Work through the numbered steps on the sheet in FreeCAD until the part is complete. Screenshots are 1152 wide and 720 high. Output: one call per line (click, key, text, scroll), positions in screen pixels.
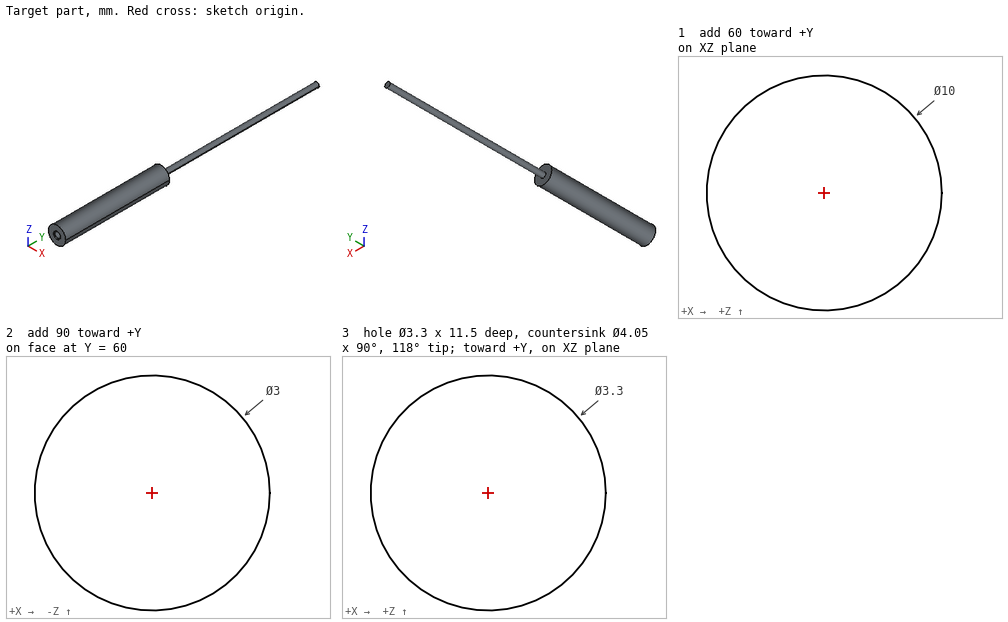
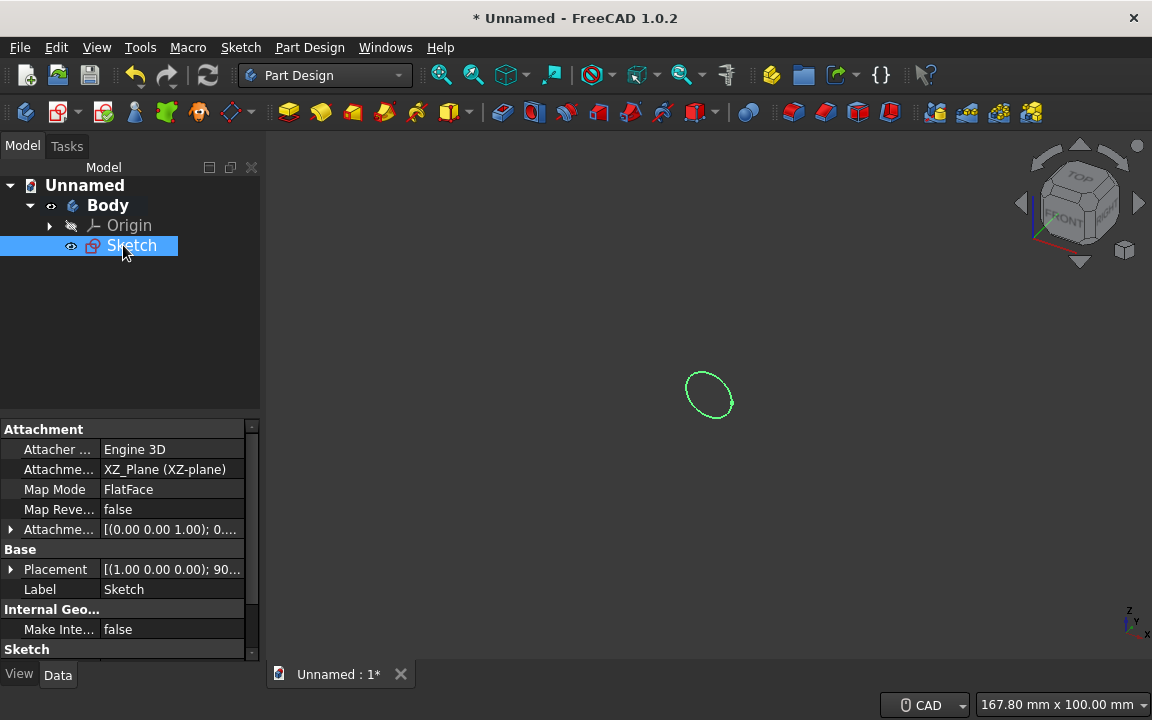
click(290, 112)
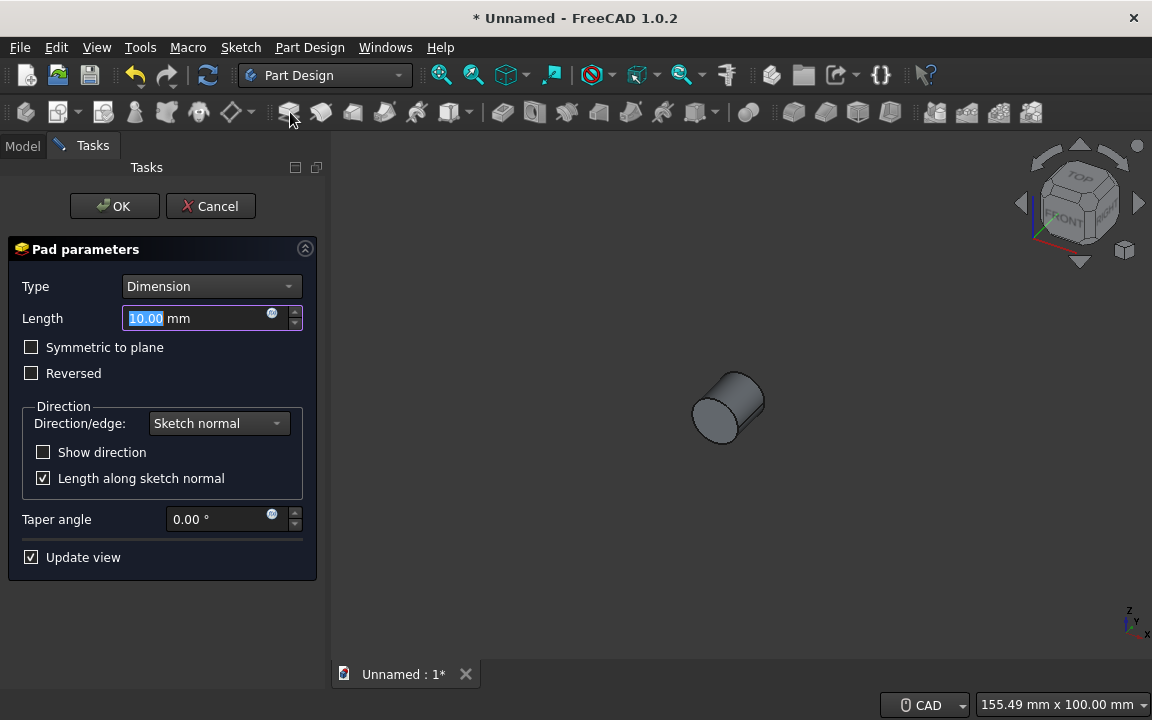
text(60)
key(Tab)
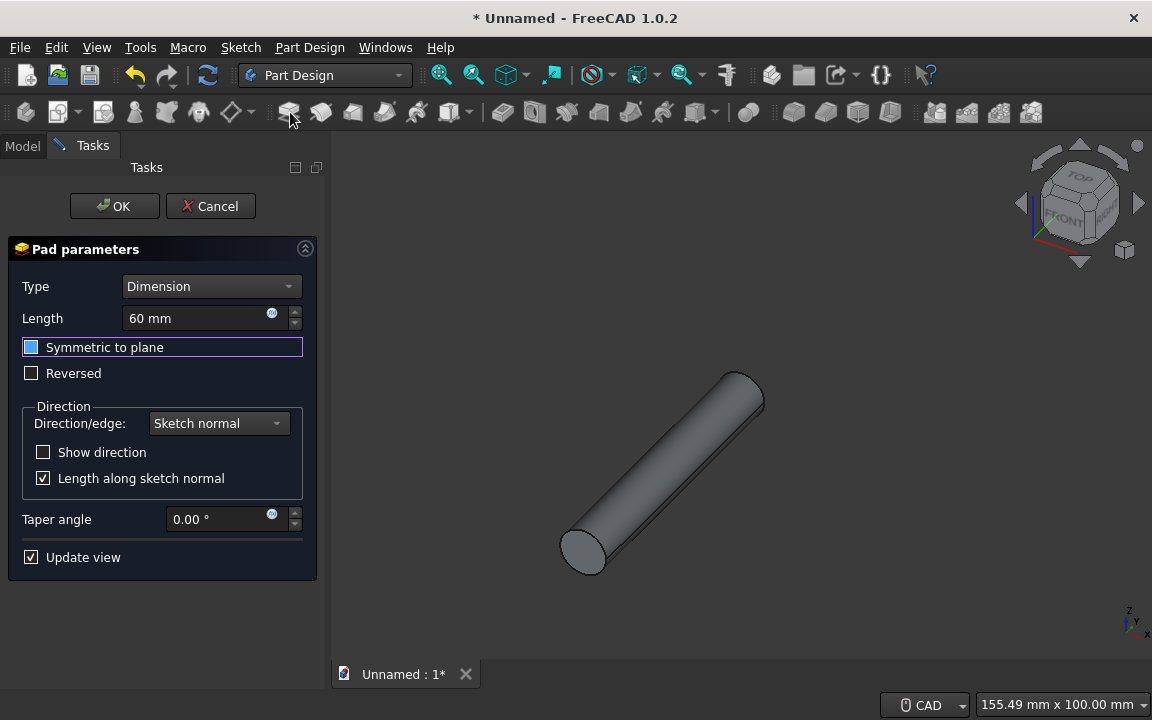
click(30, 373)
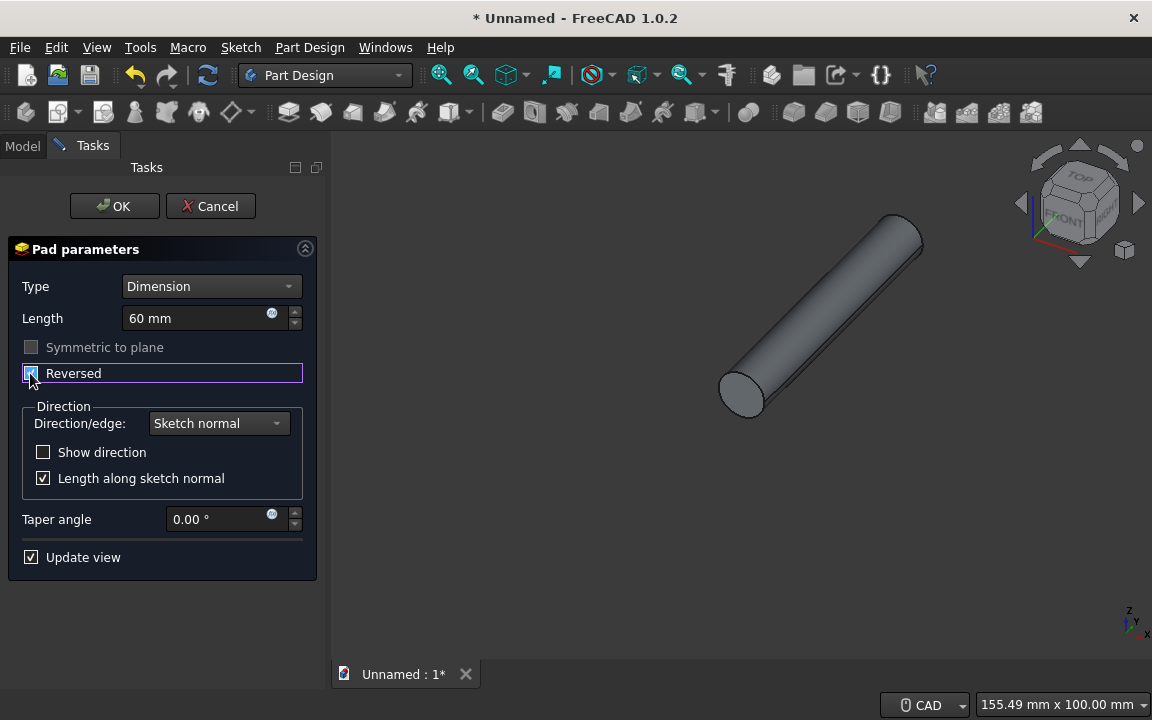
click(115, 206)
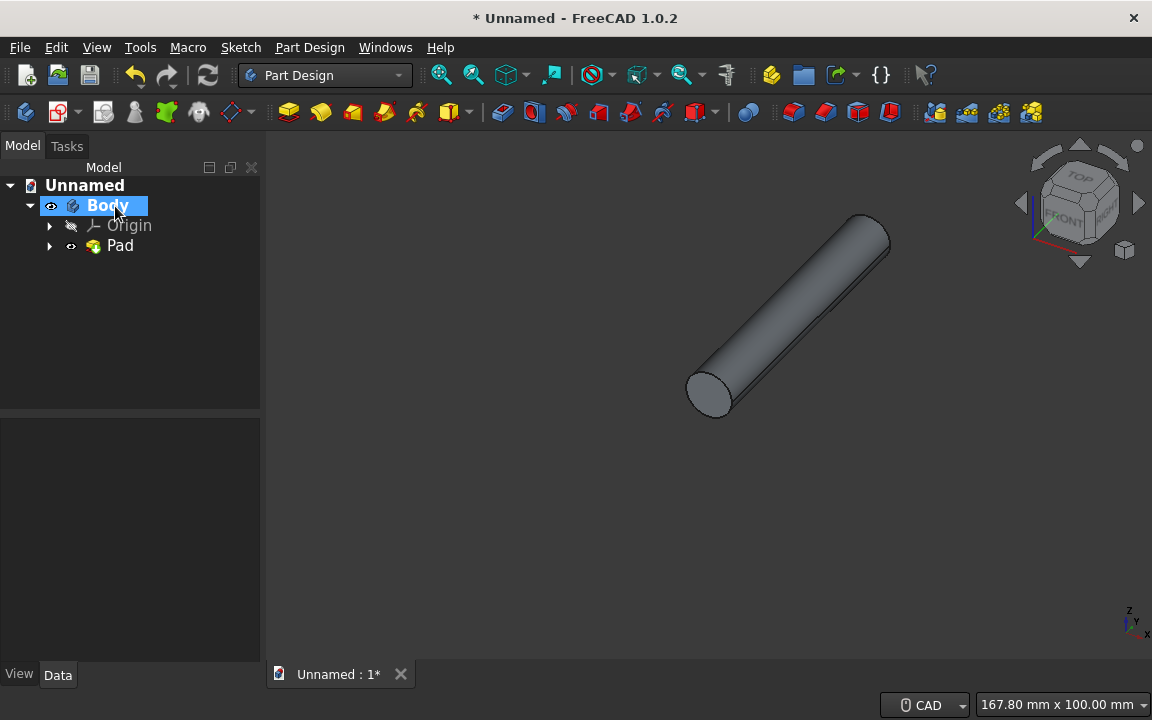
click(442, 76)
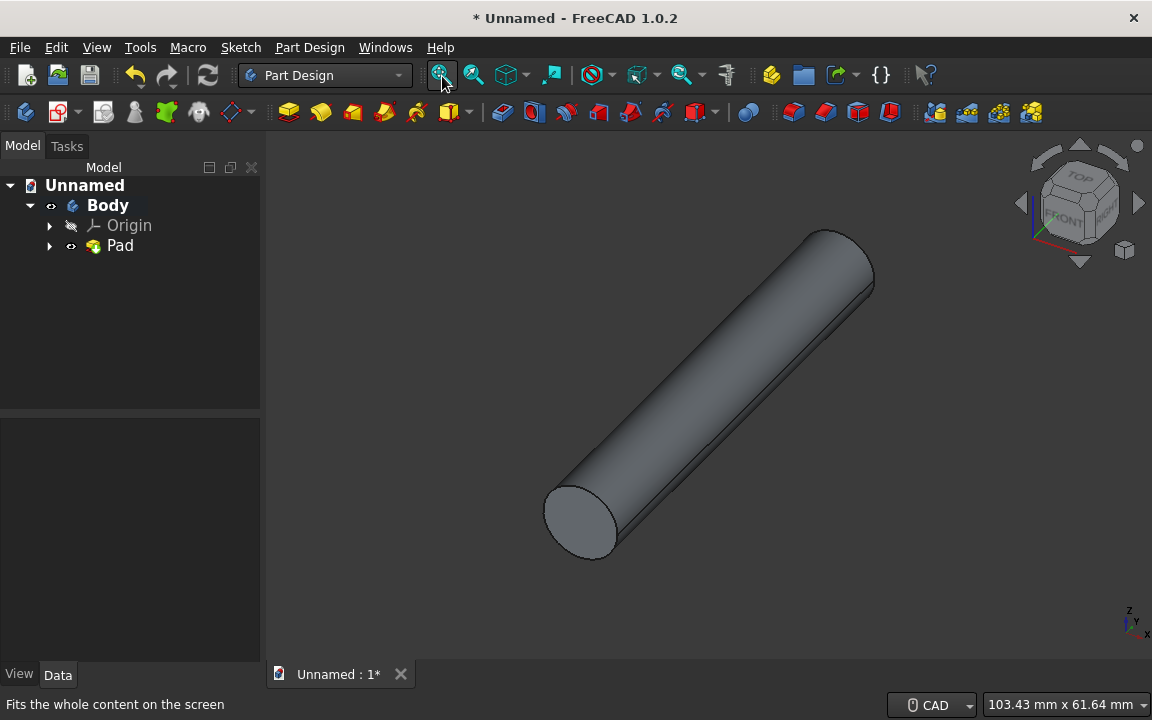
key(4)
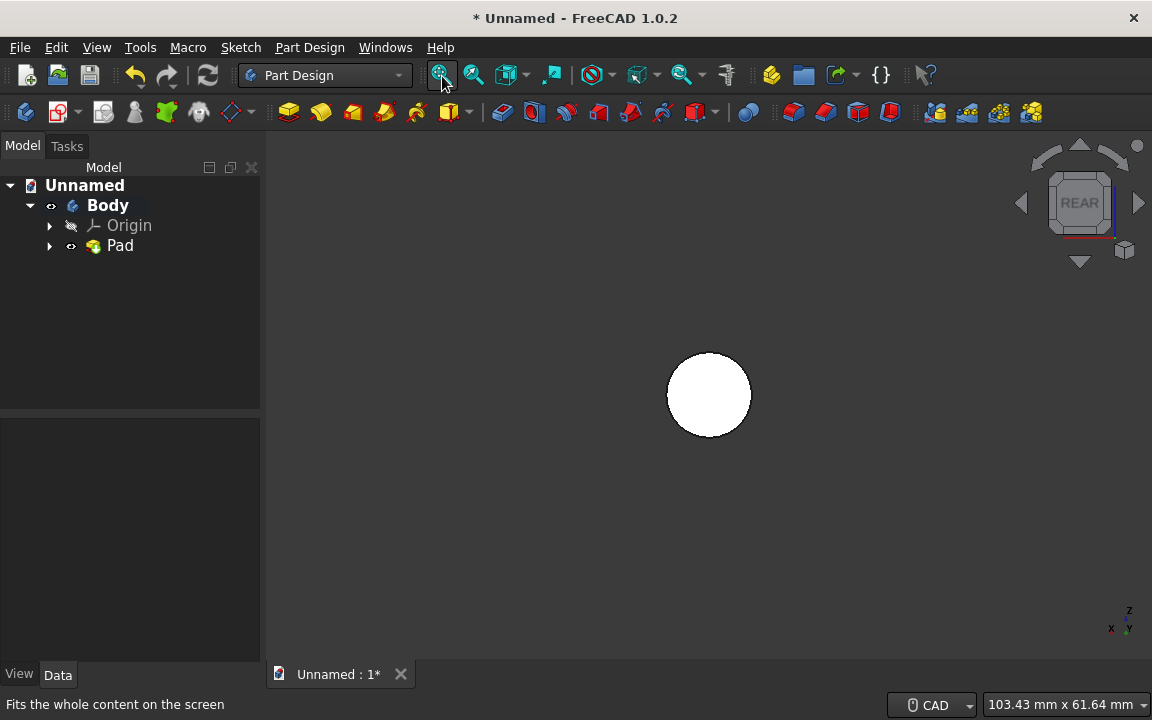
click(442, 76)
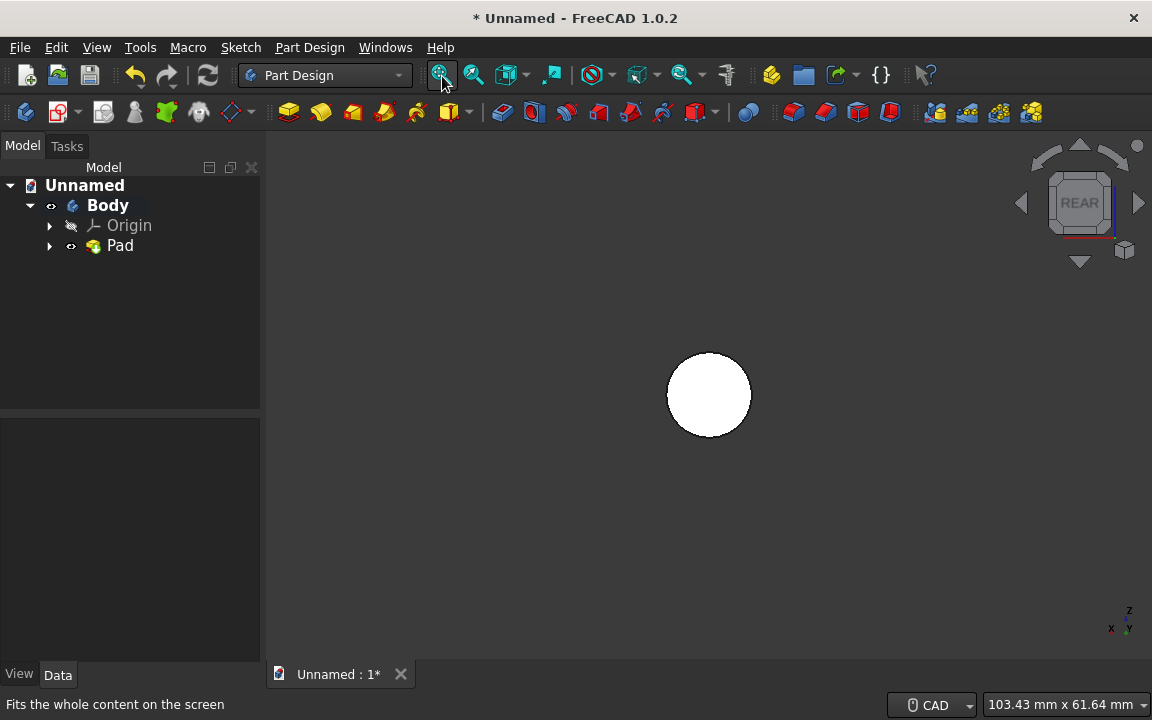
click(709, 394)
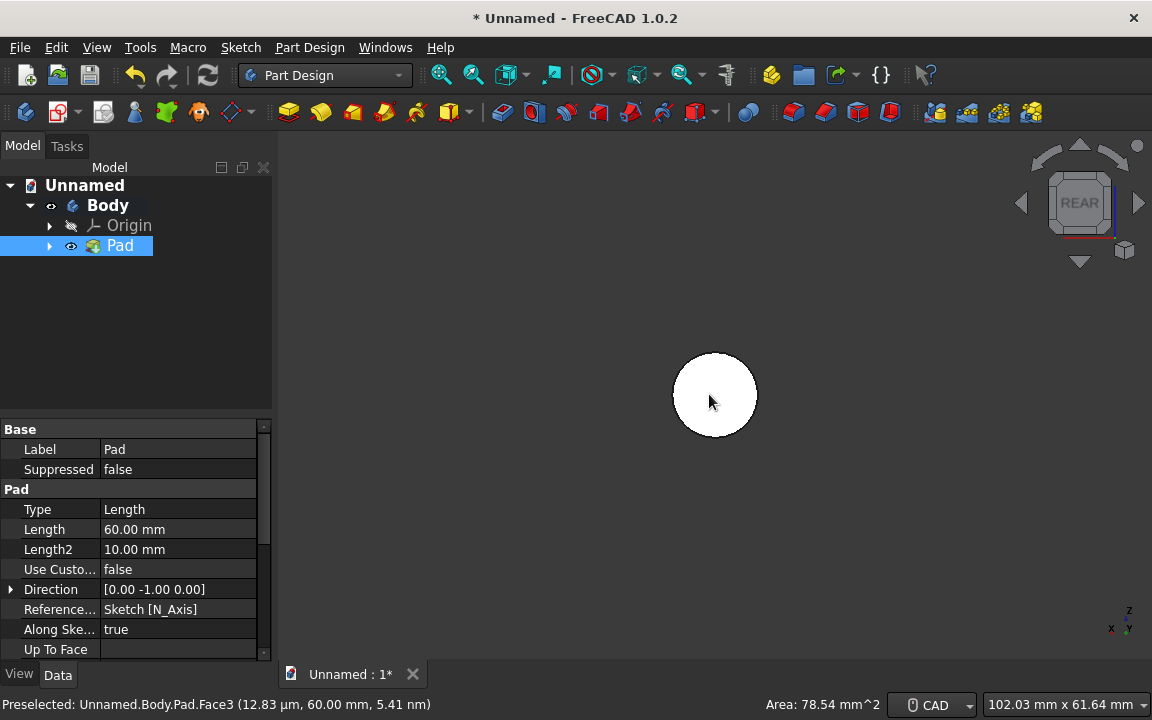
click(58, 112)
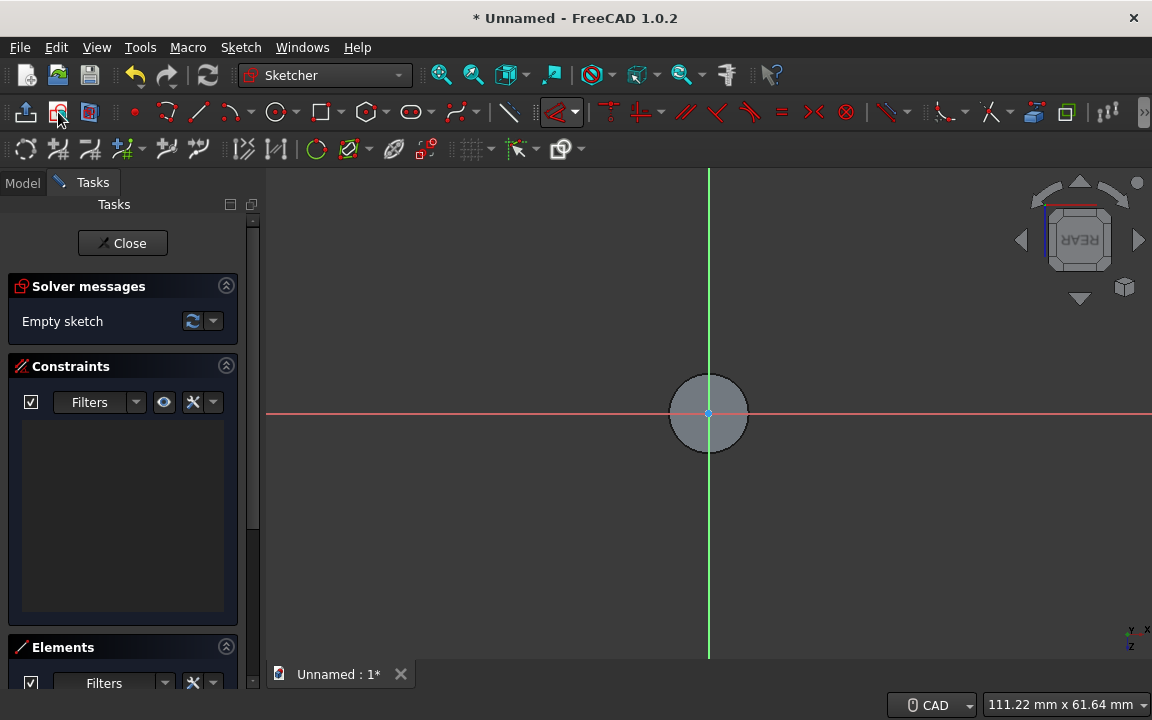
scroll(714, 413, up, 13)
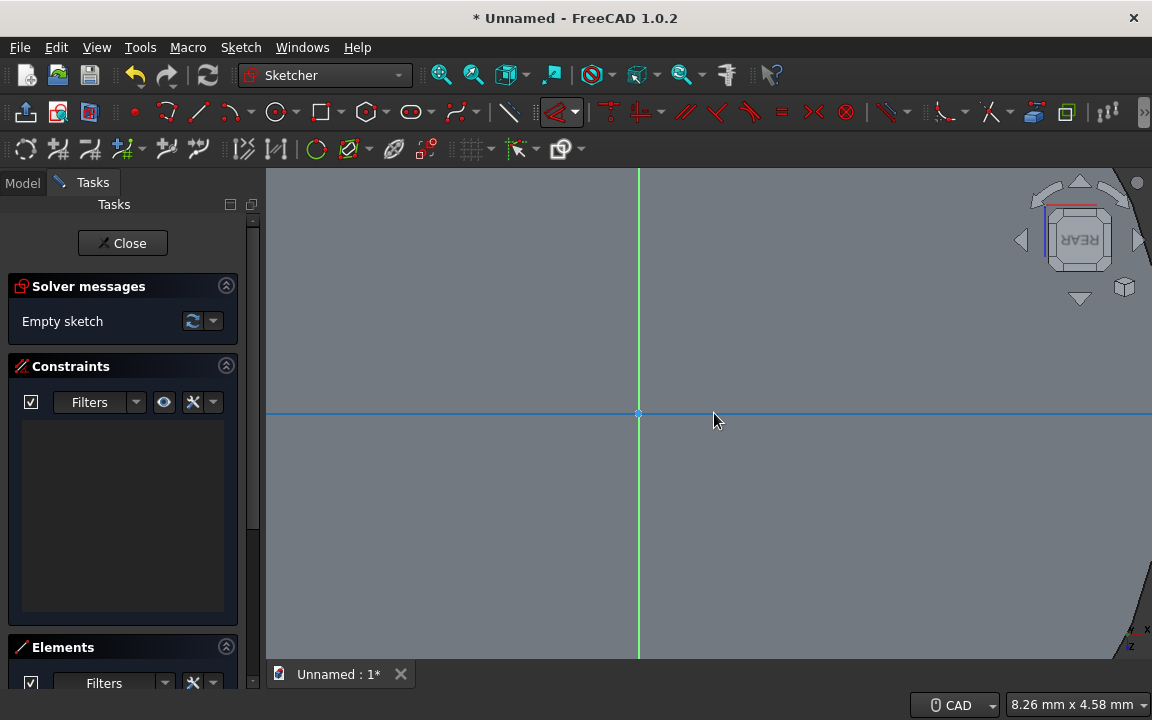
click(276, 112)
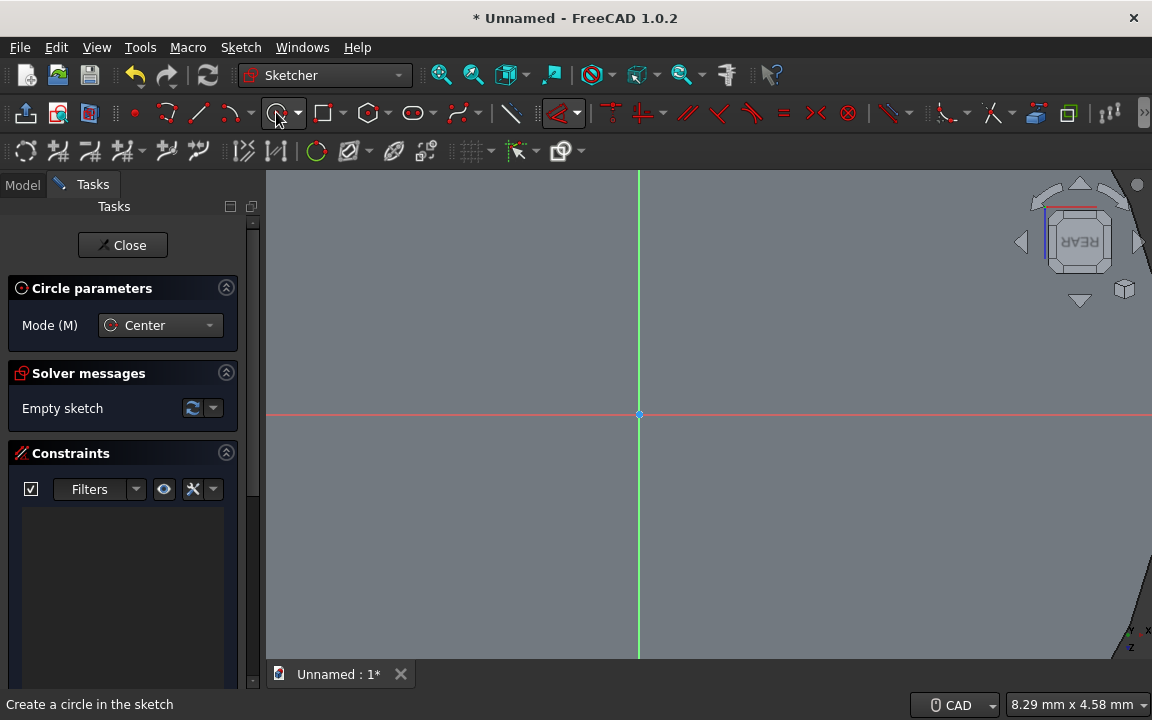
click(639, 414)
click(753, 301)
key(Escape)